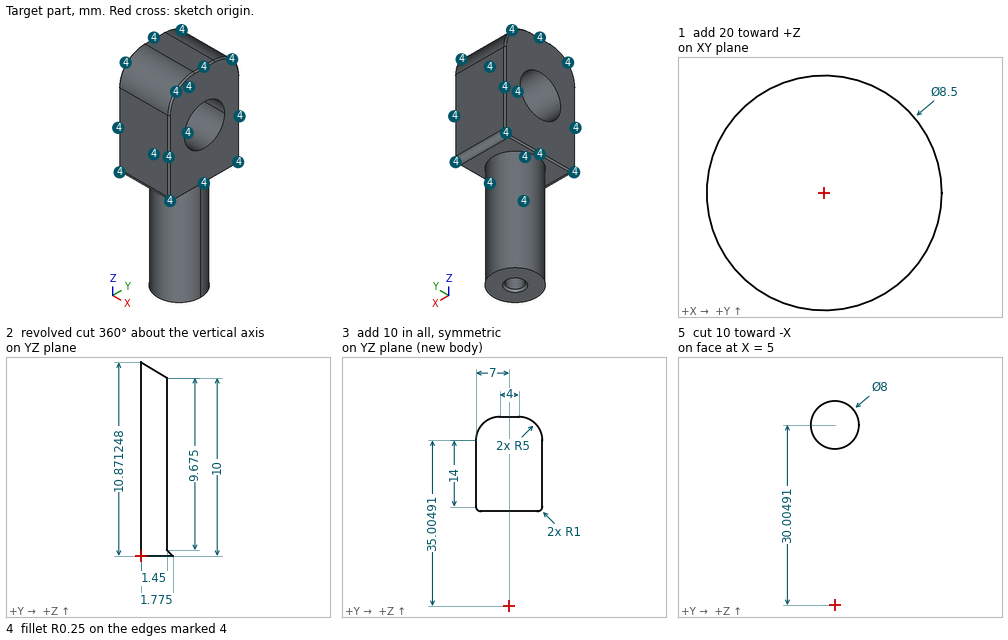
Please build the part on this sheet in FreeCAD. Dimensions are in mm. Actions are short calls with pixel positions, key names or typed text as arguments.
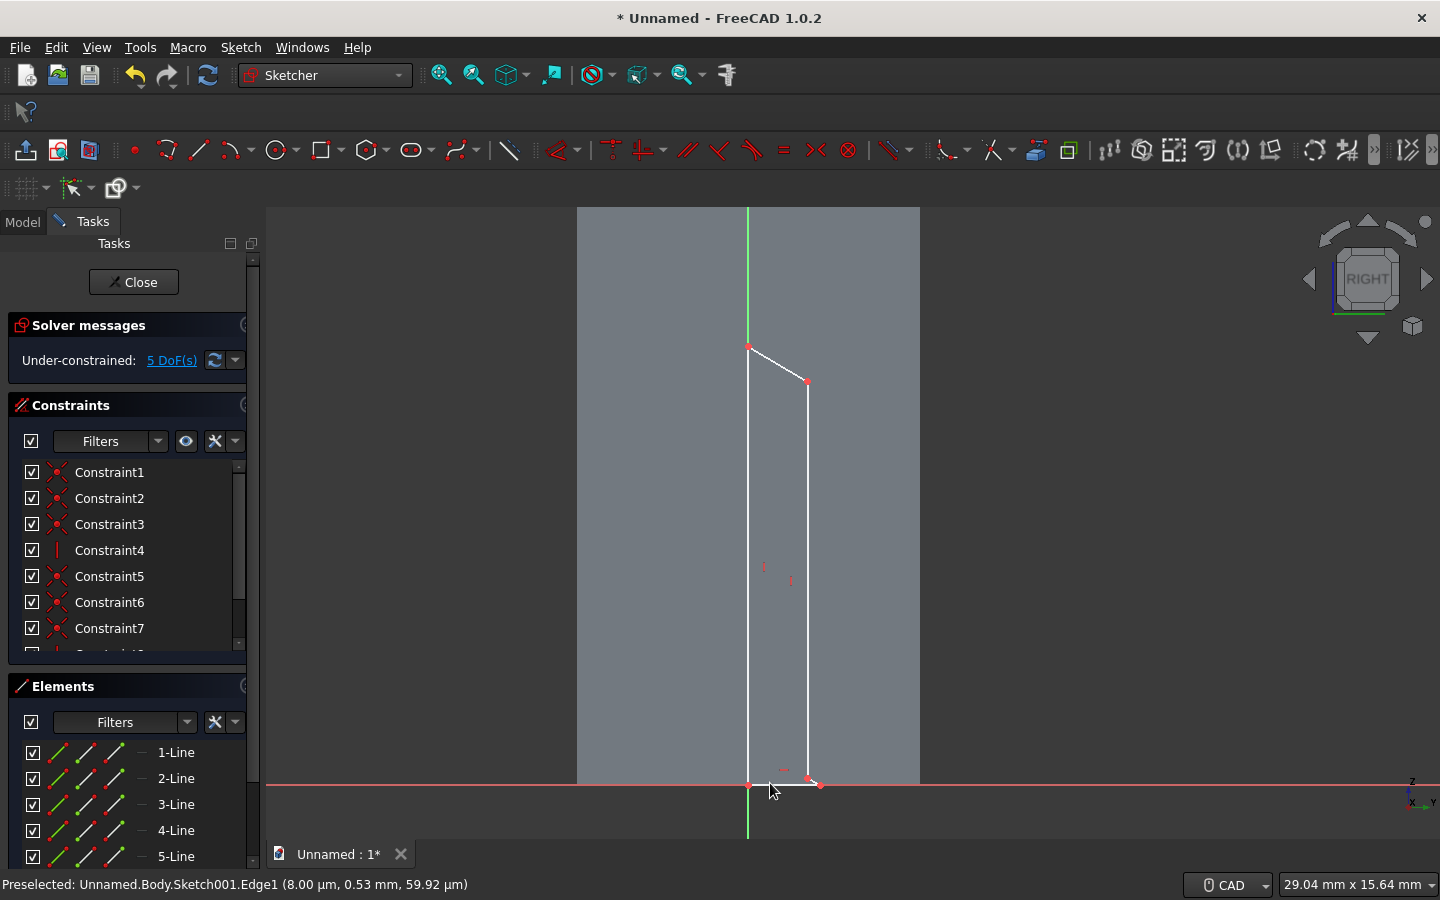
click(556, 150)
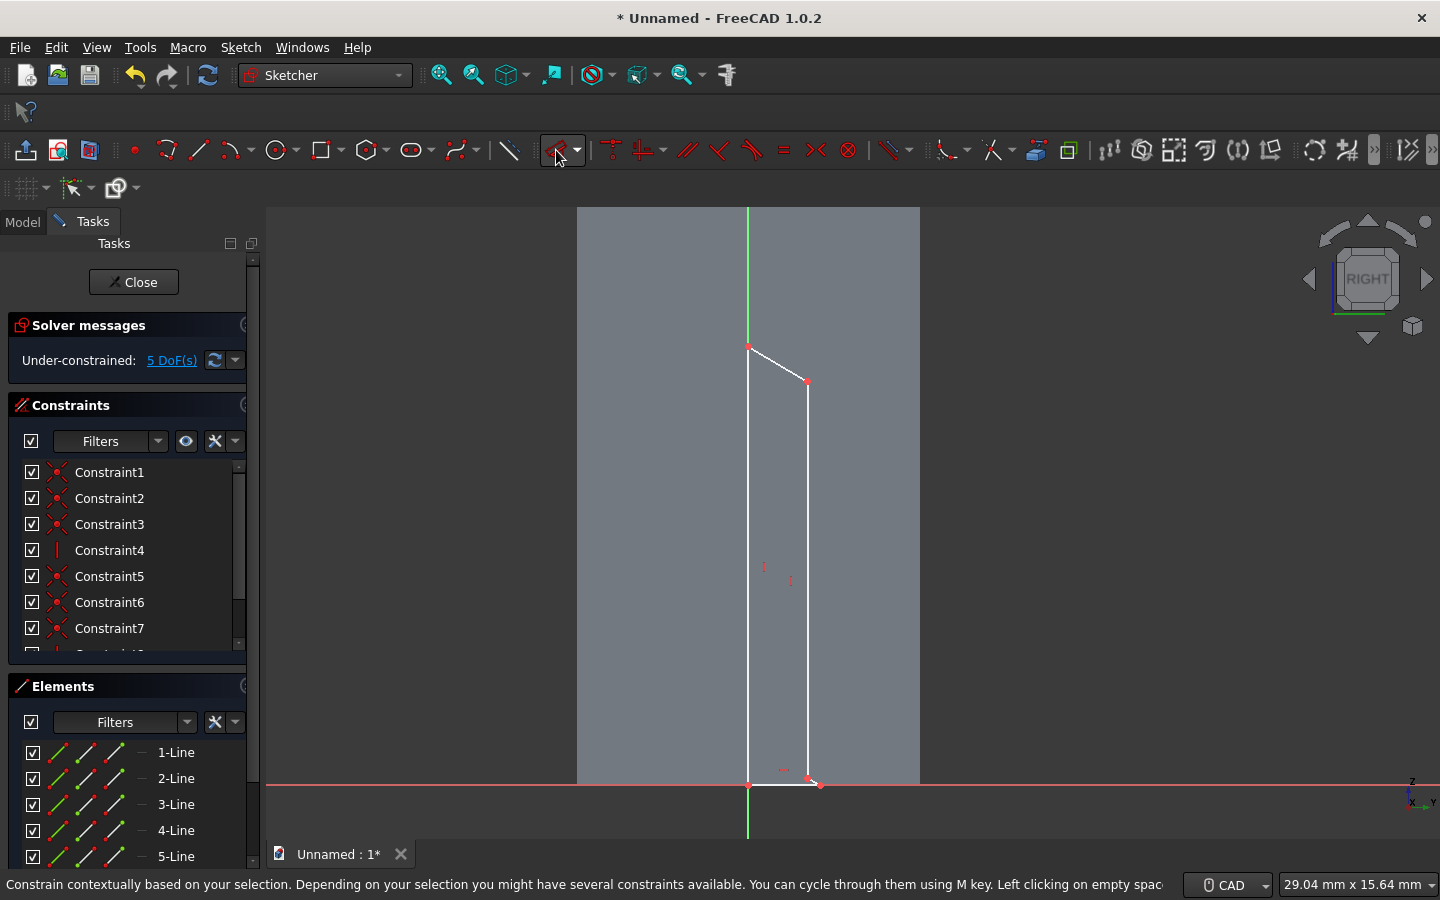
click(808, 382)
click(714, 584)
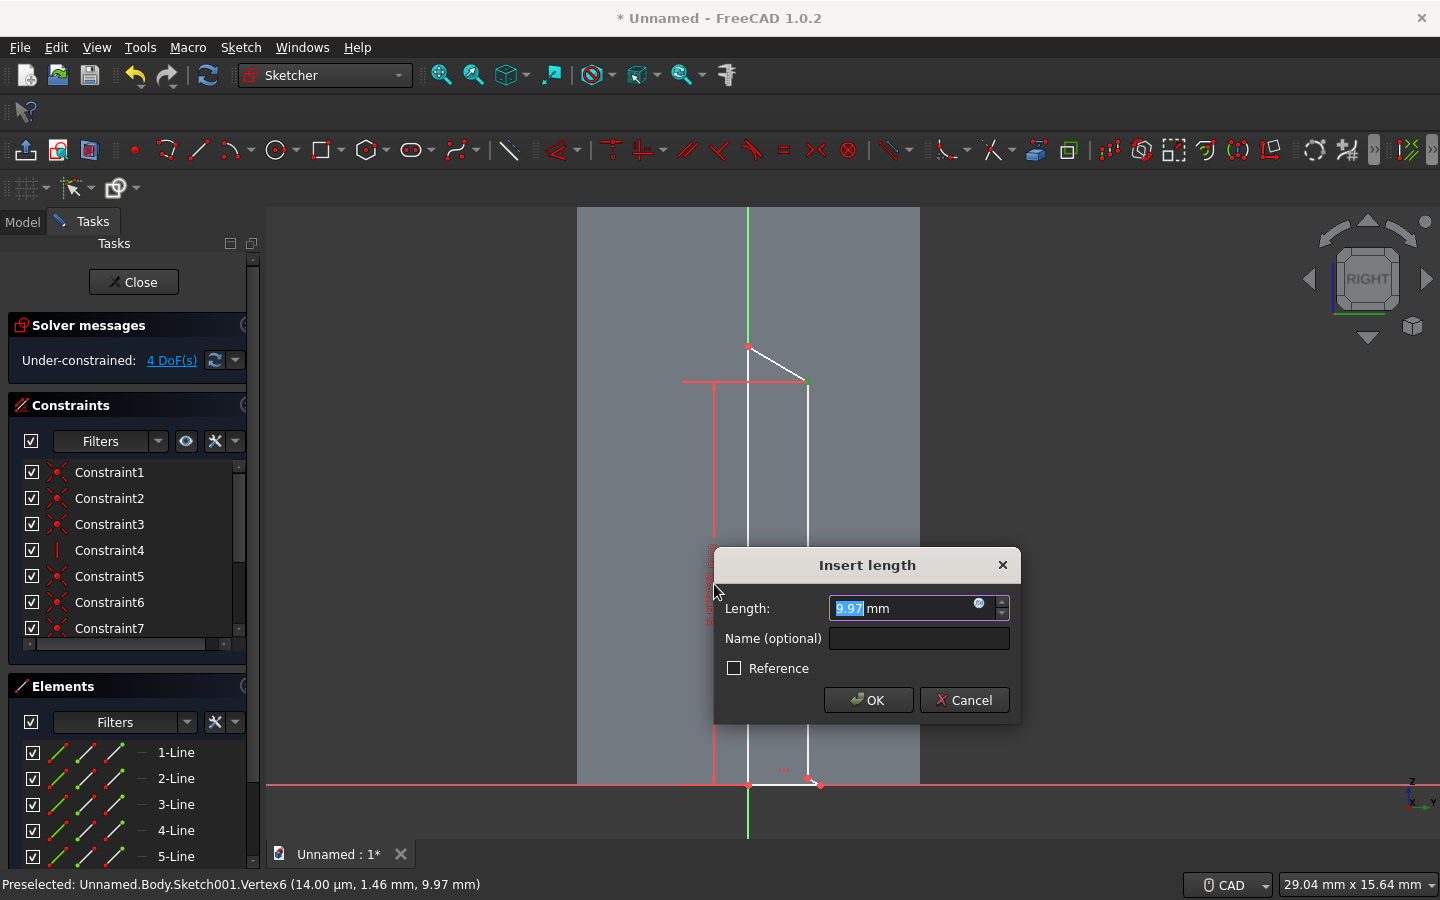
text(10)
key(Return)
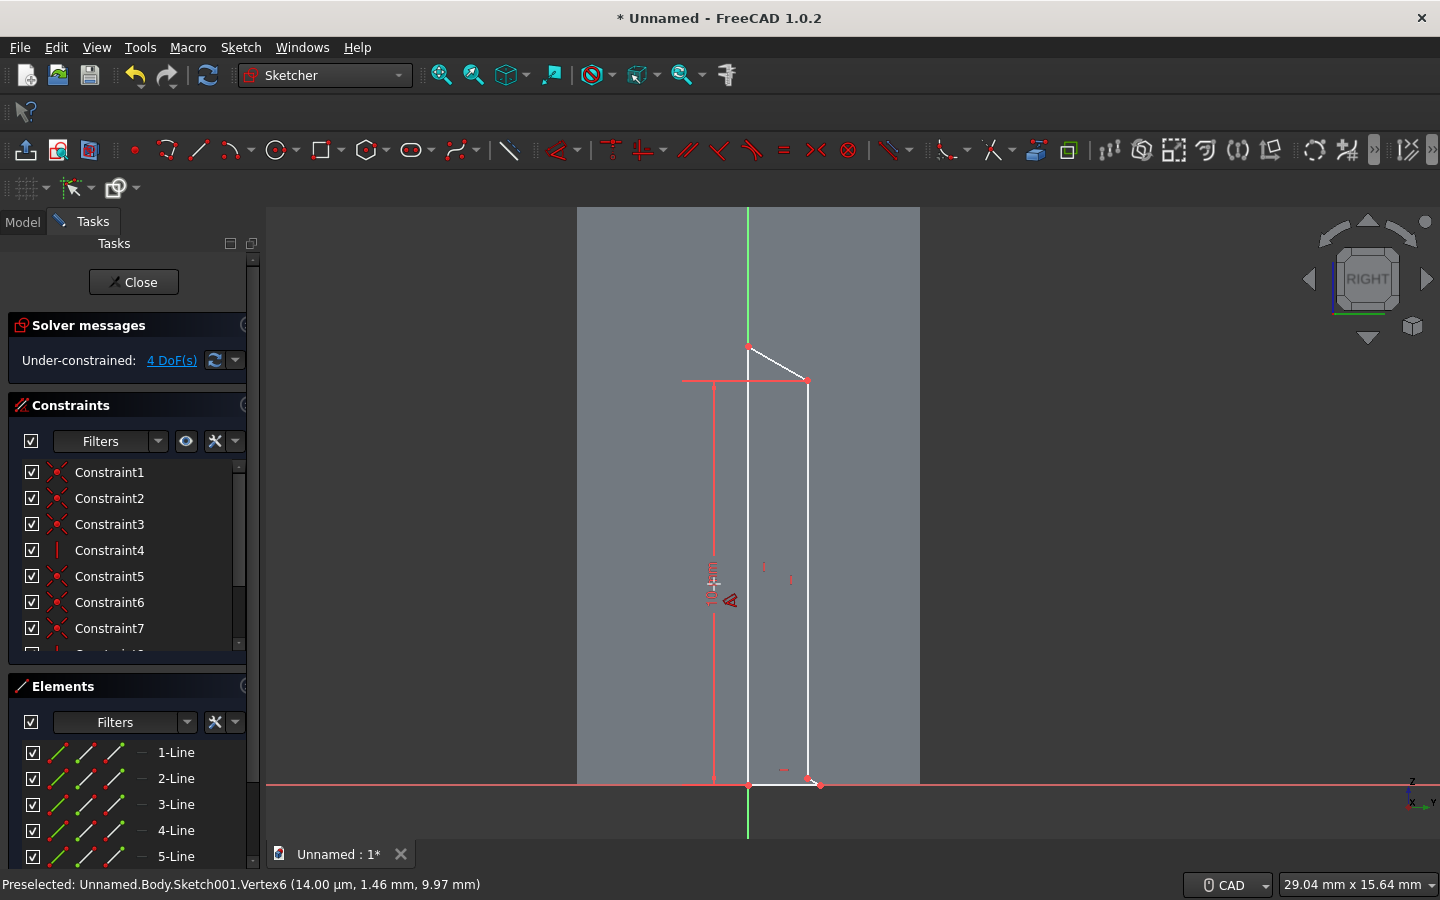
click(770, 785)
click(784, 751)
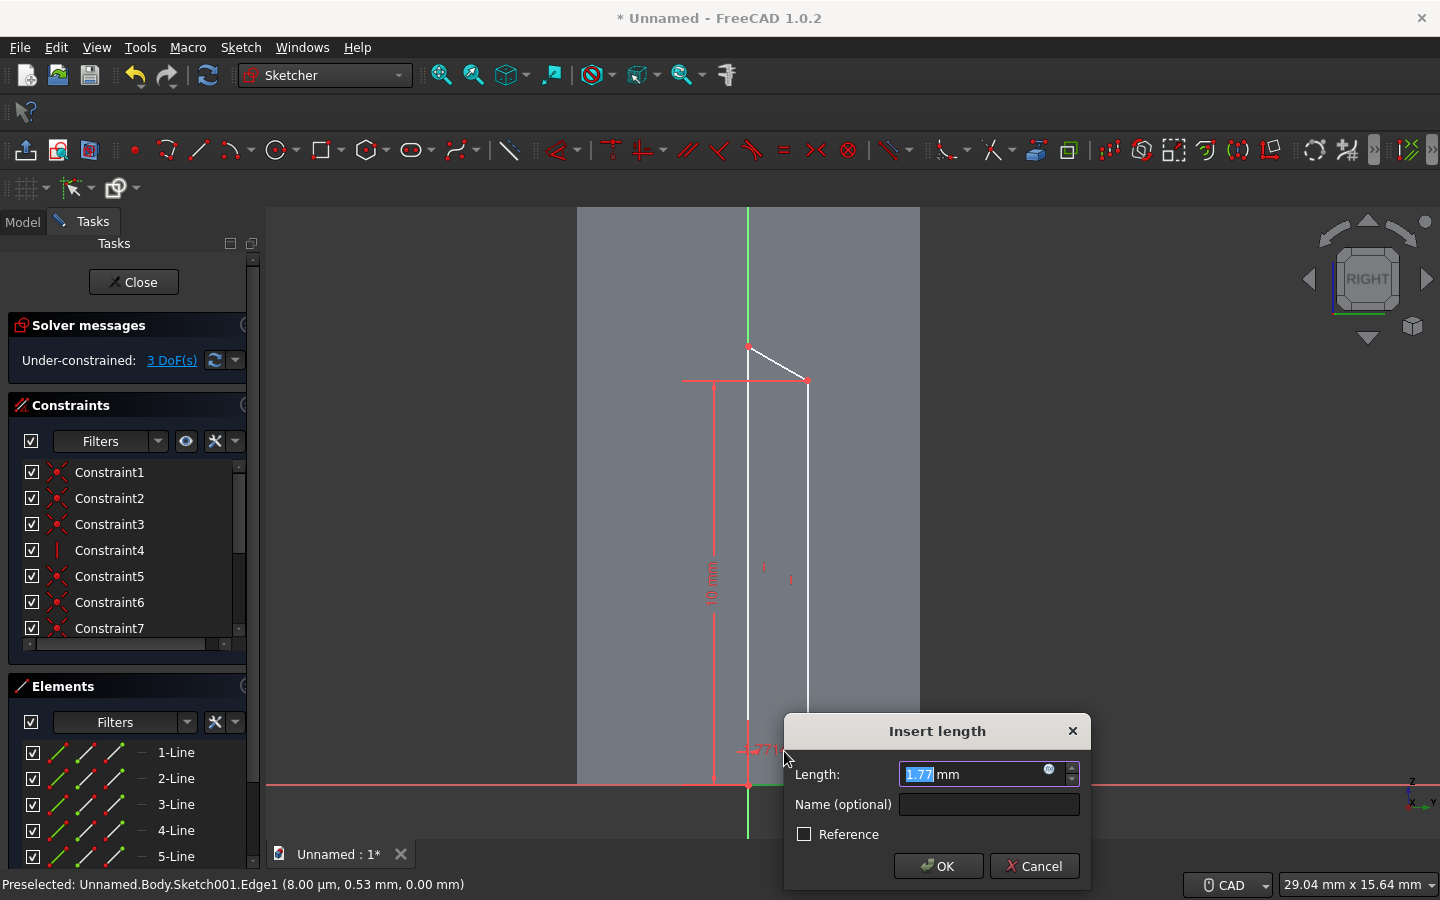
text(1.775)
key(Return)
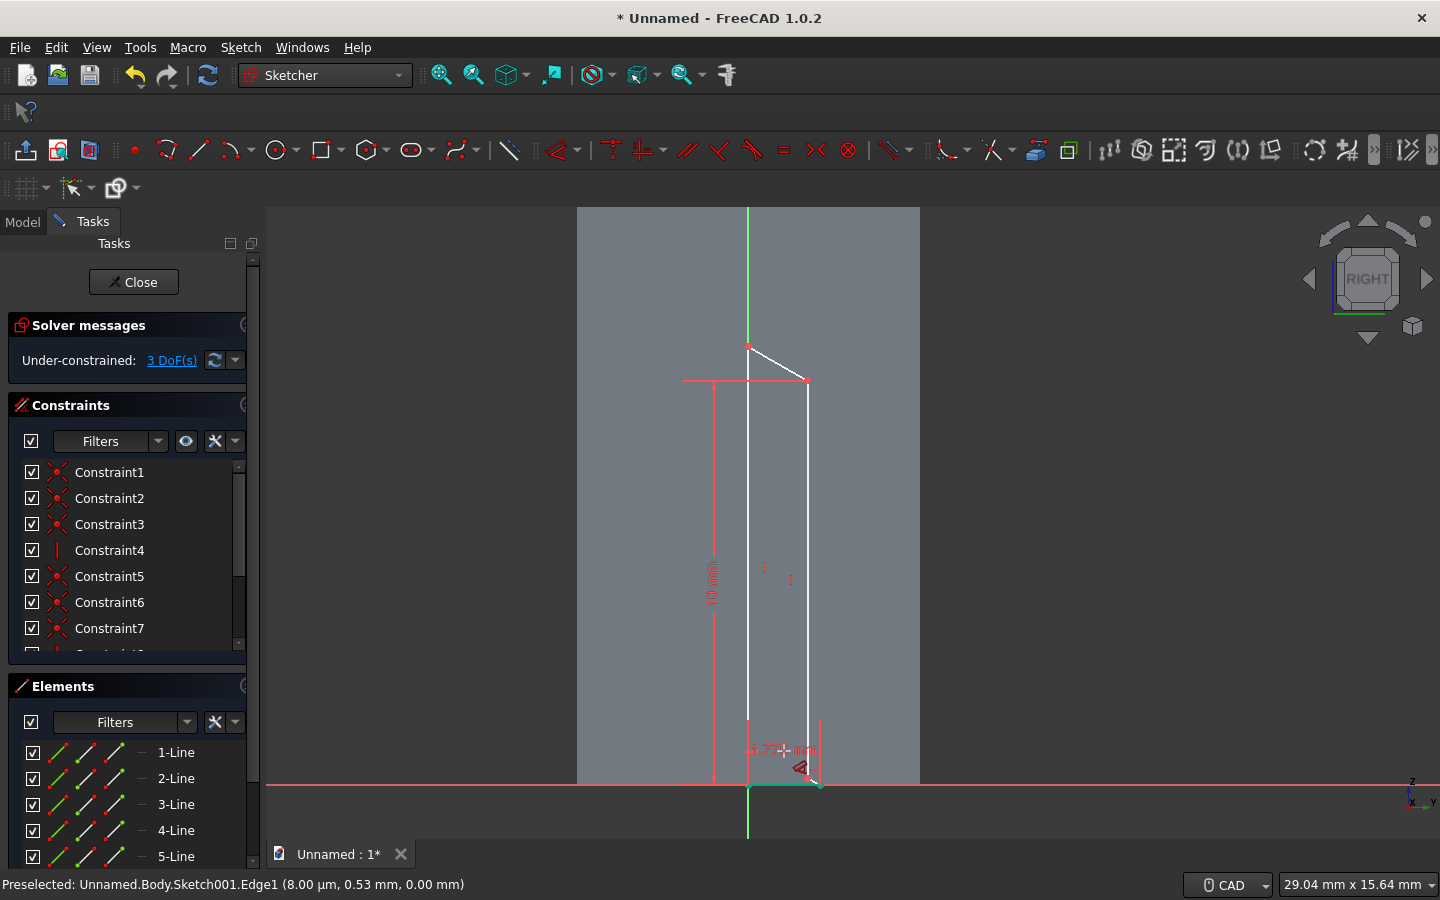
click(808, 659)
click(842, 580)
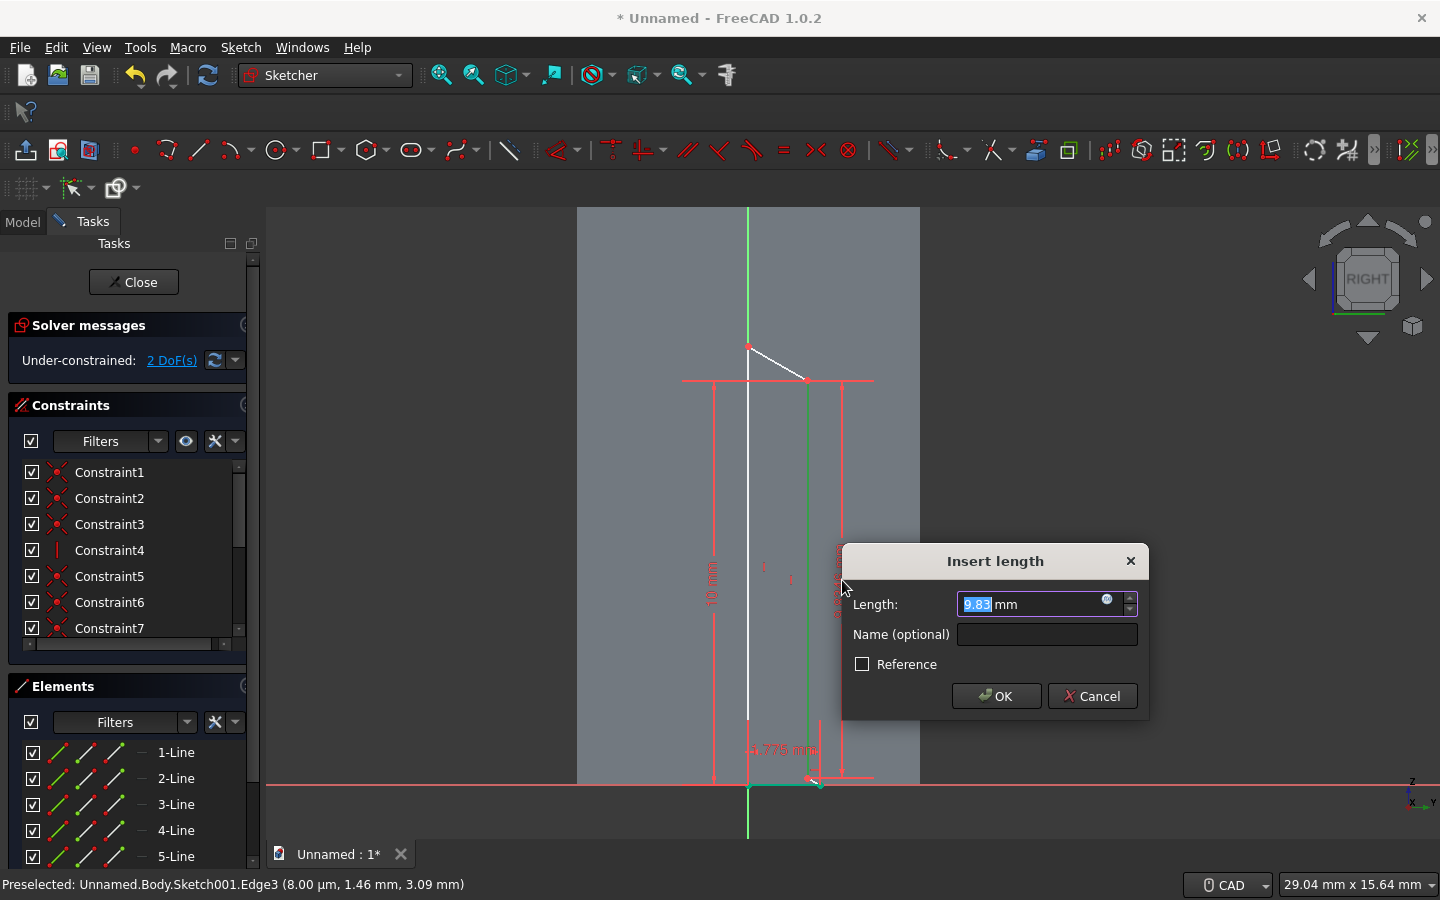
text(9.675)
key(Return)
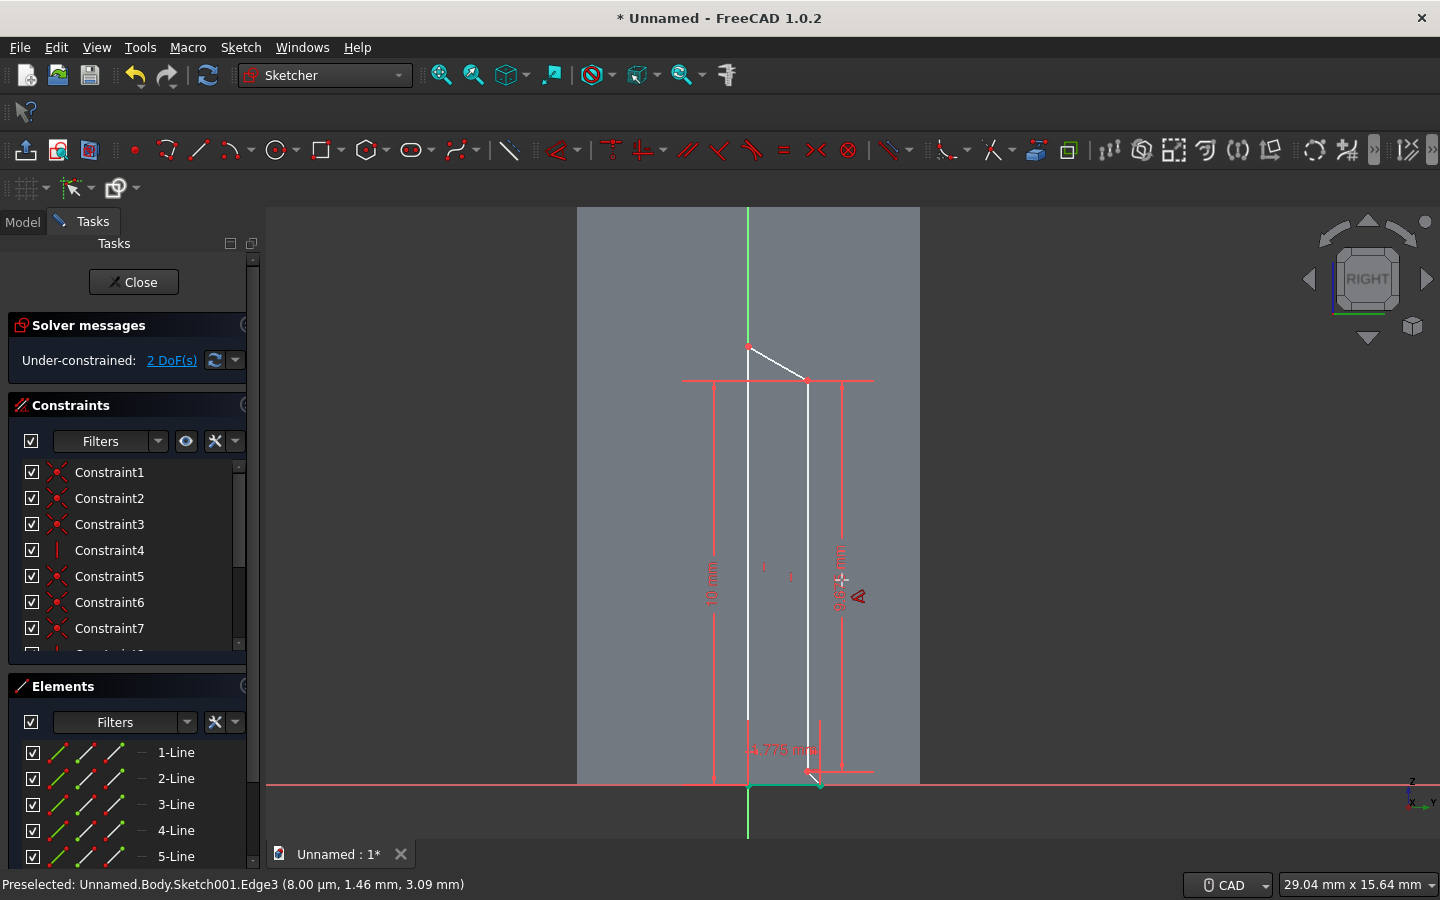
click(808, 772)
click(778, 714)